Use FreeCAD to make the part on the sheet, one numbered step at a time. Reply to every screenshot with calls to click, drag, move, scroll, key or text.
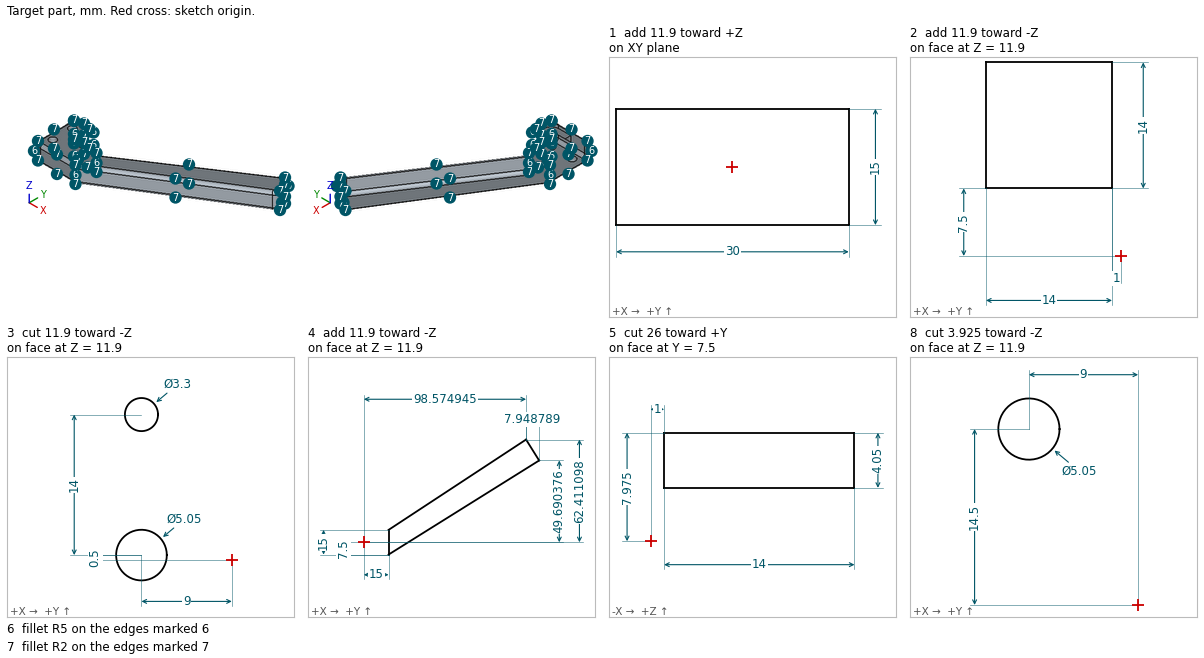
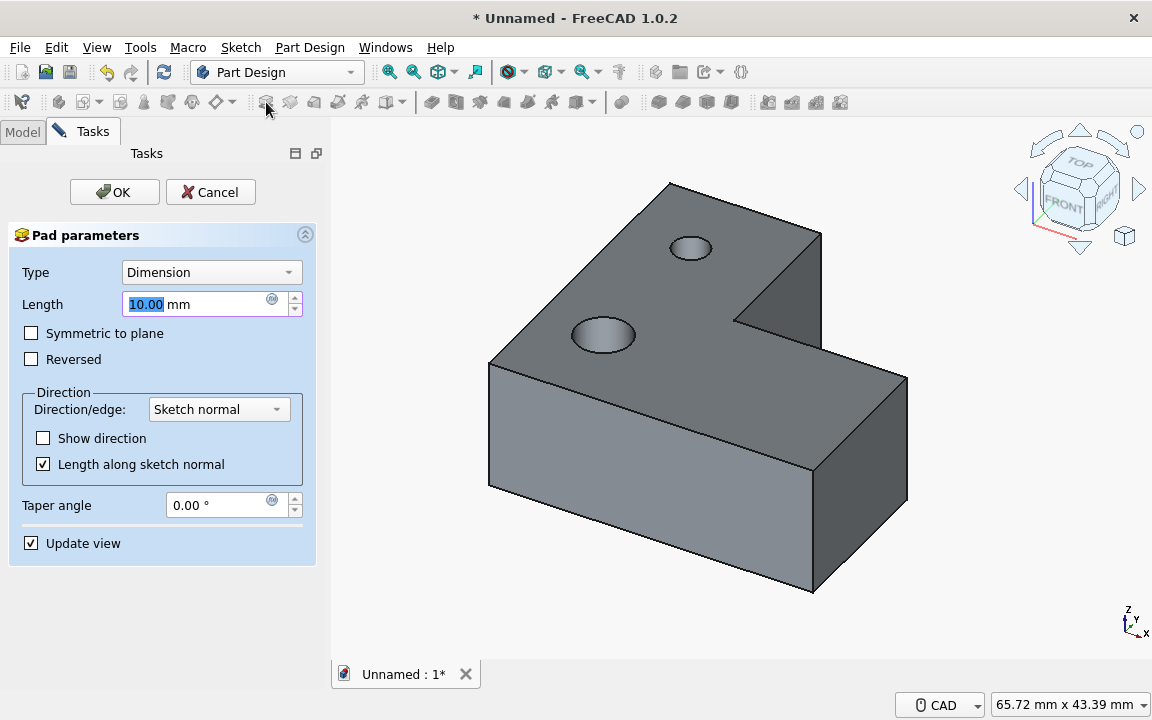
text(11.9)
key(Tab)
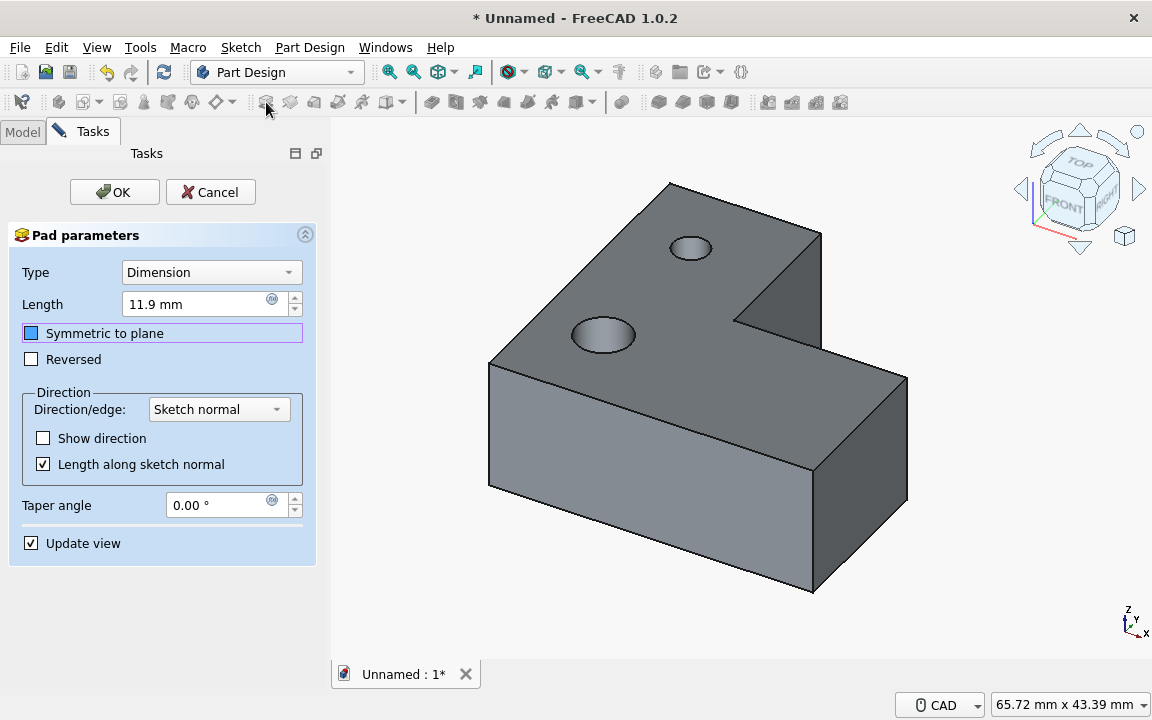
click(30, 359)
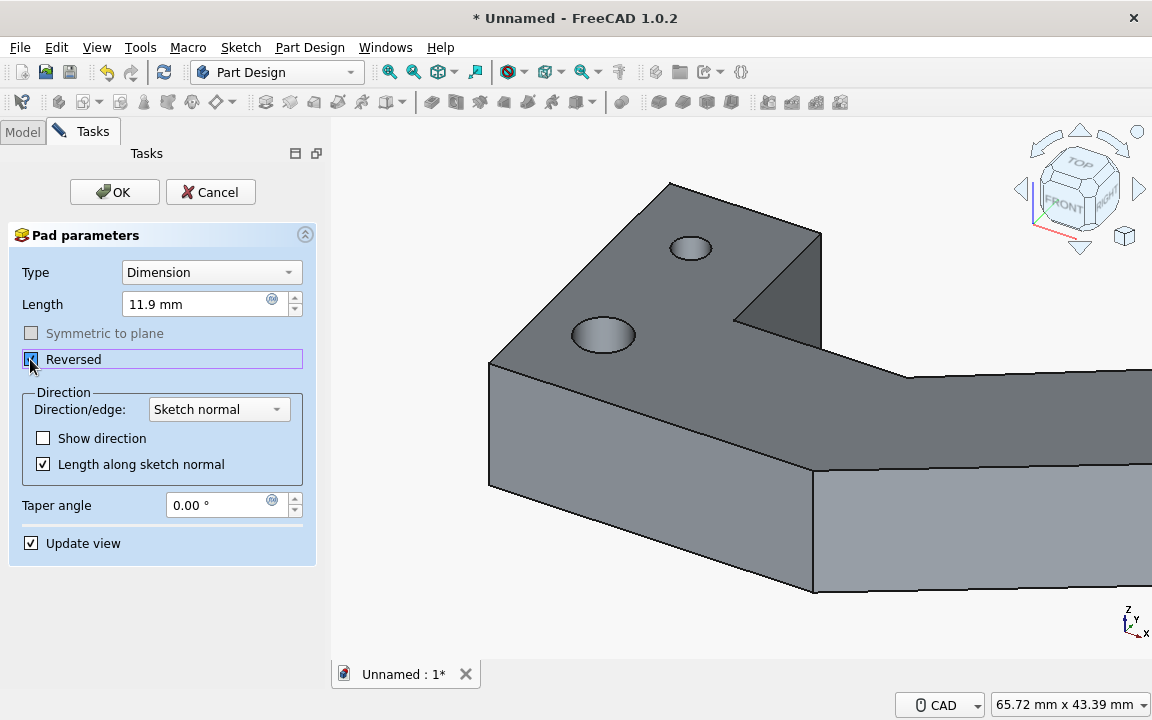
click(115, 192)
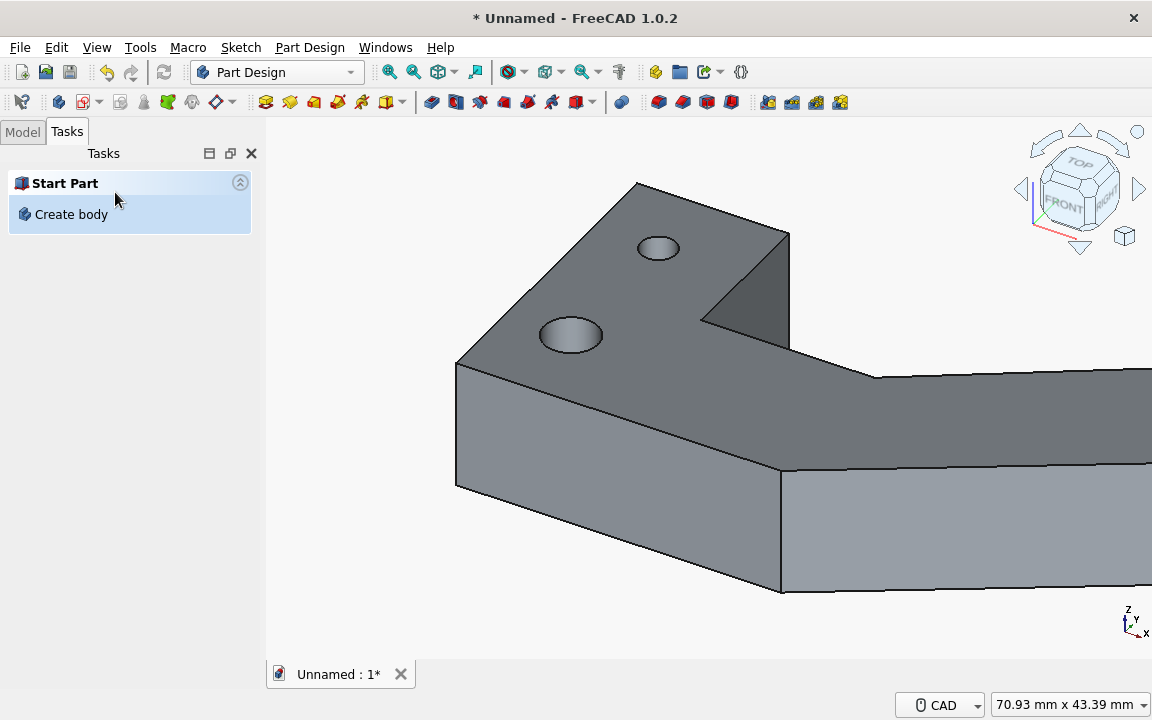
click(390, 72)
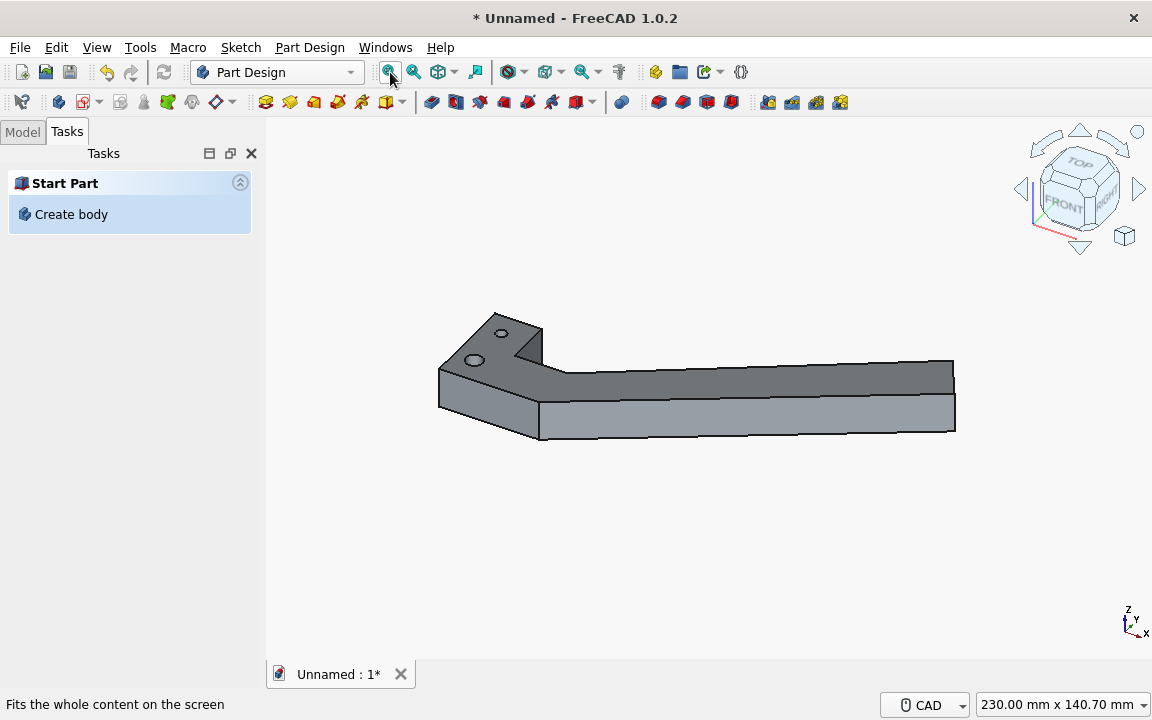
key(4)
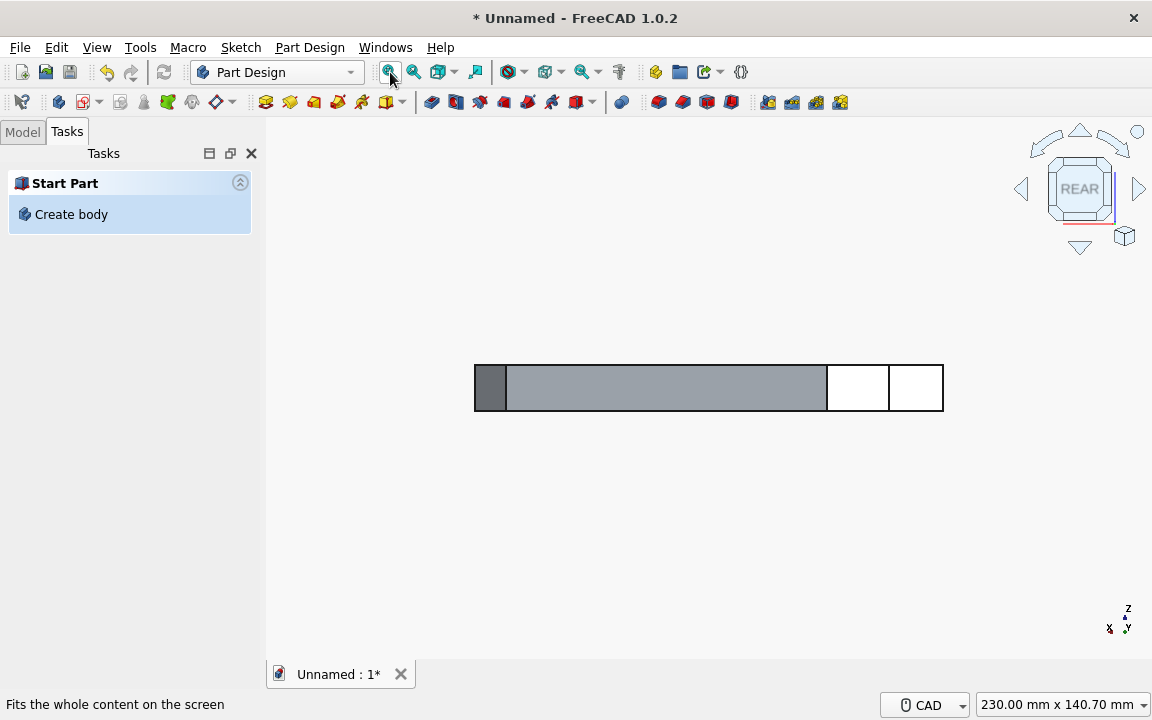
click(858, 387)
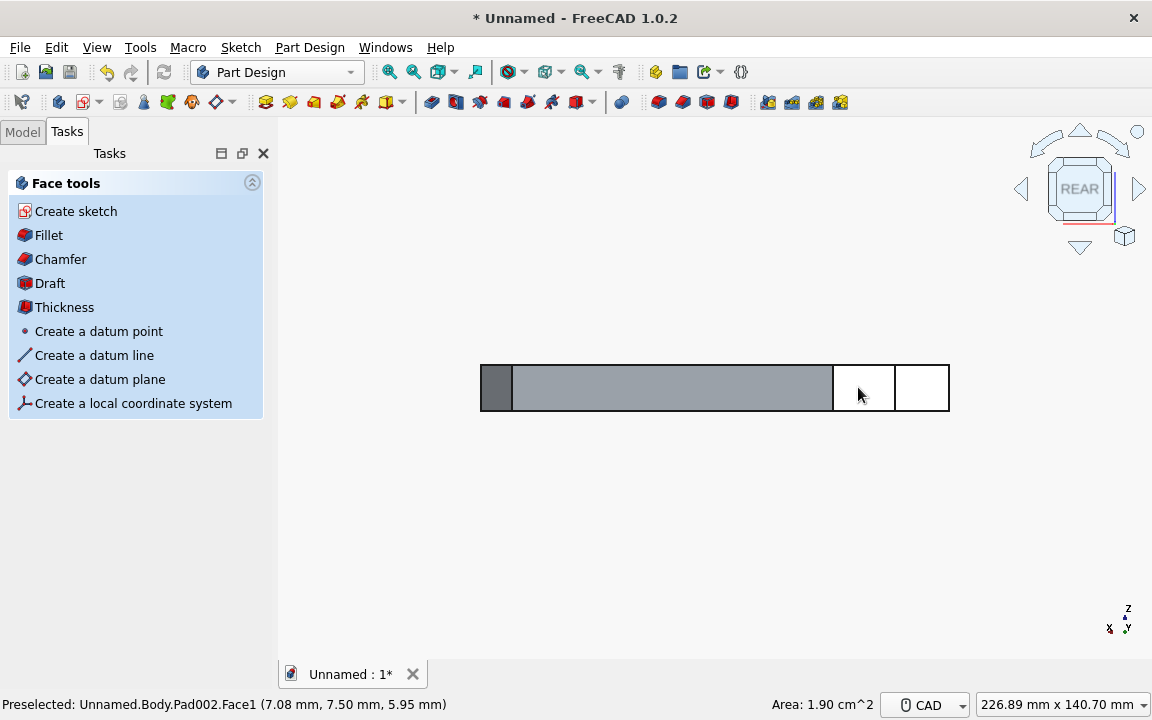
click(84, 102)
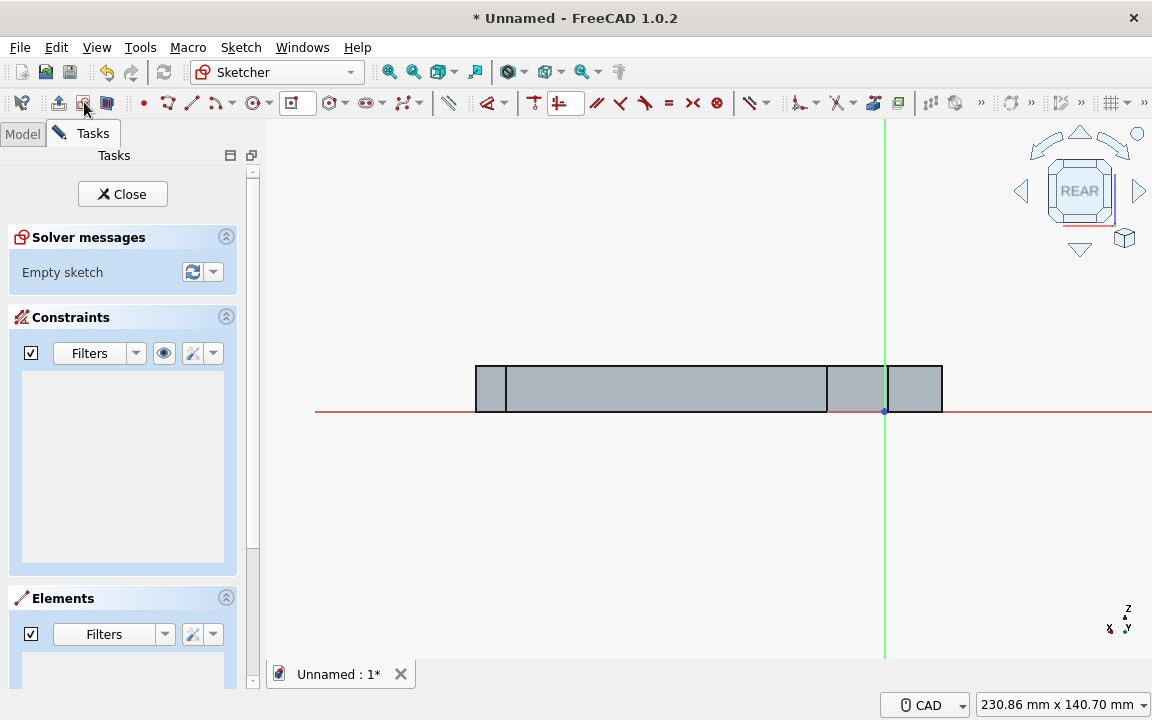
click(108, 104)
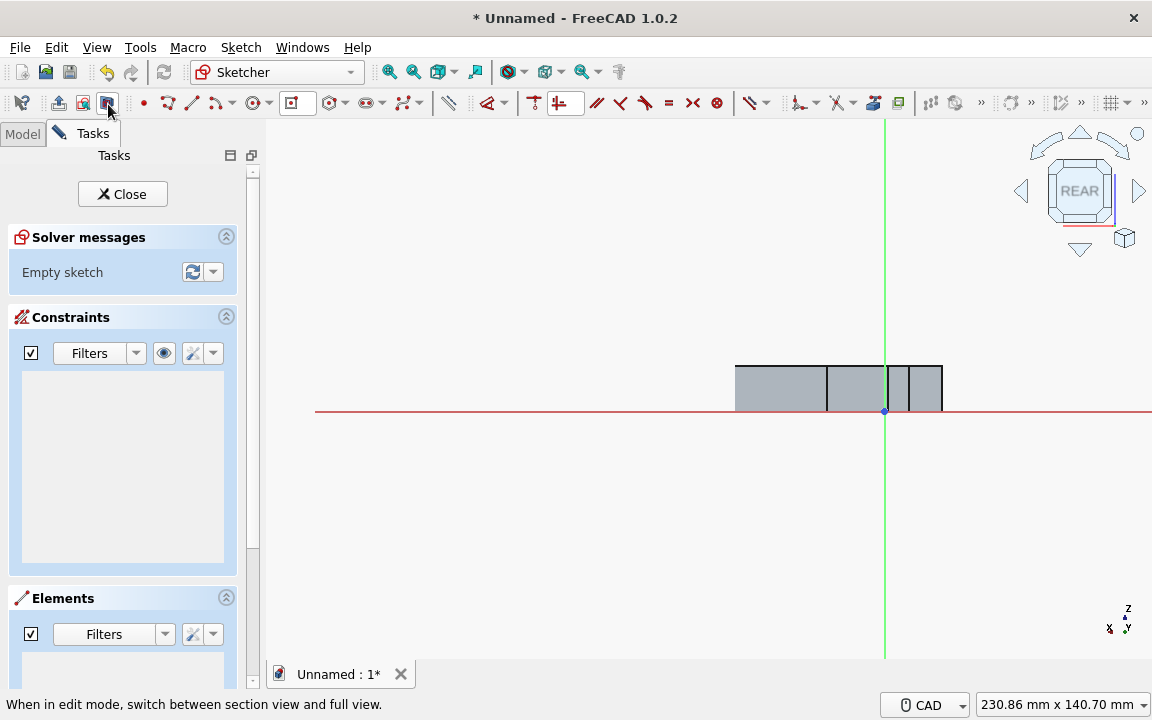
scroll(947, 397, up, 11)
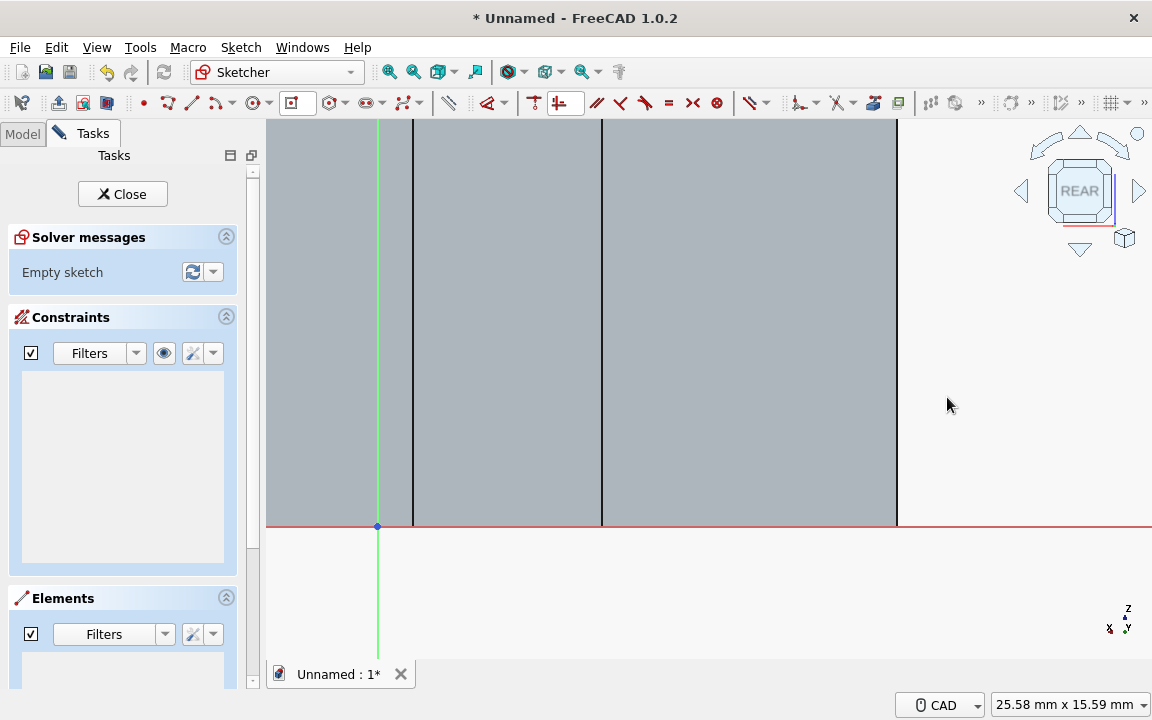
click(310, 104)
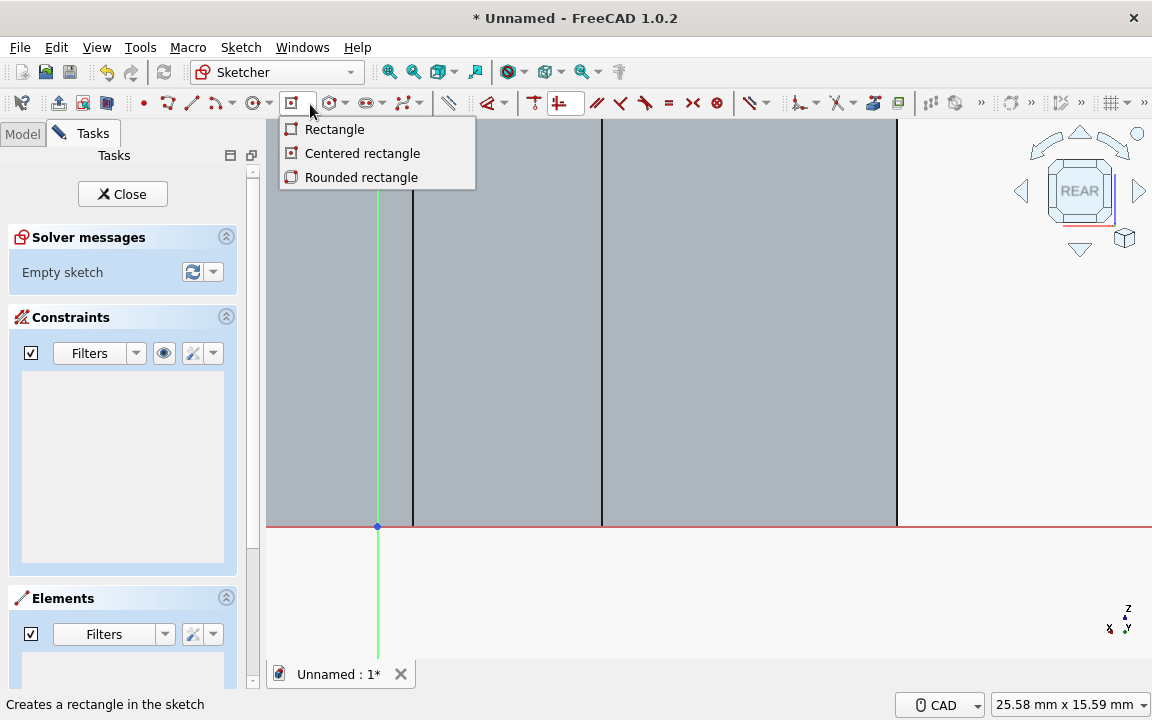
click(378, 129)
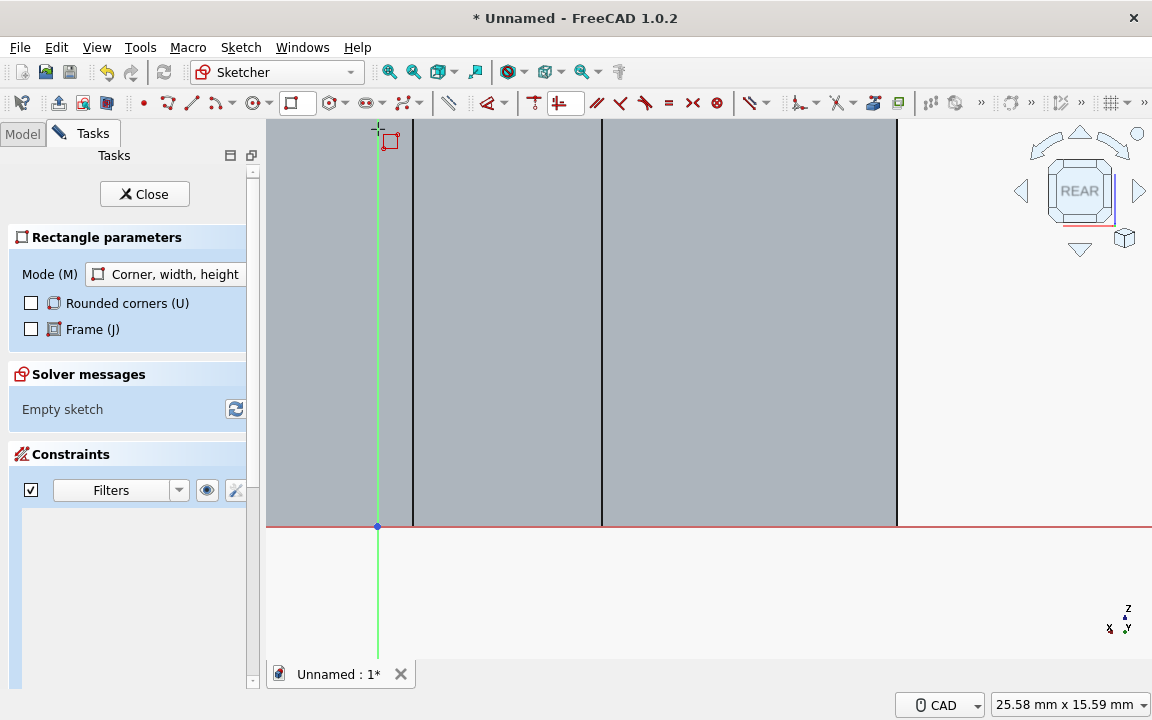
click(413, 251)
move(897, 391)